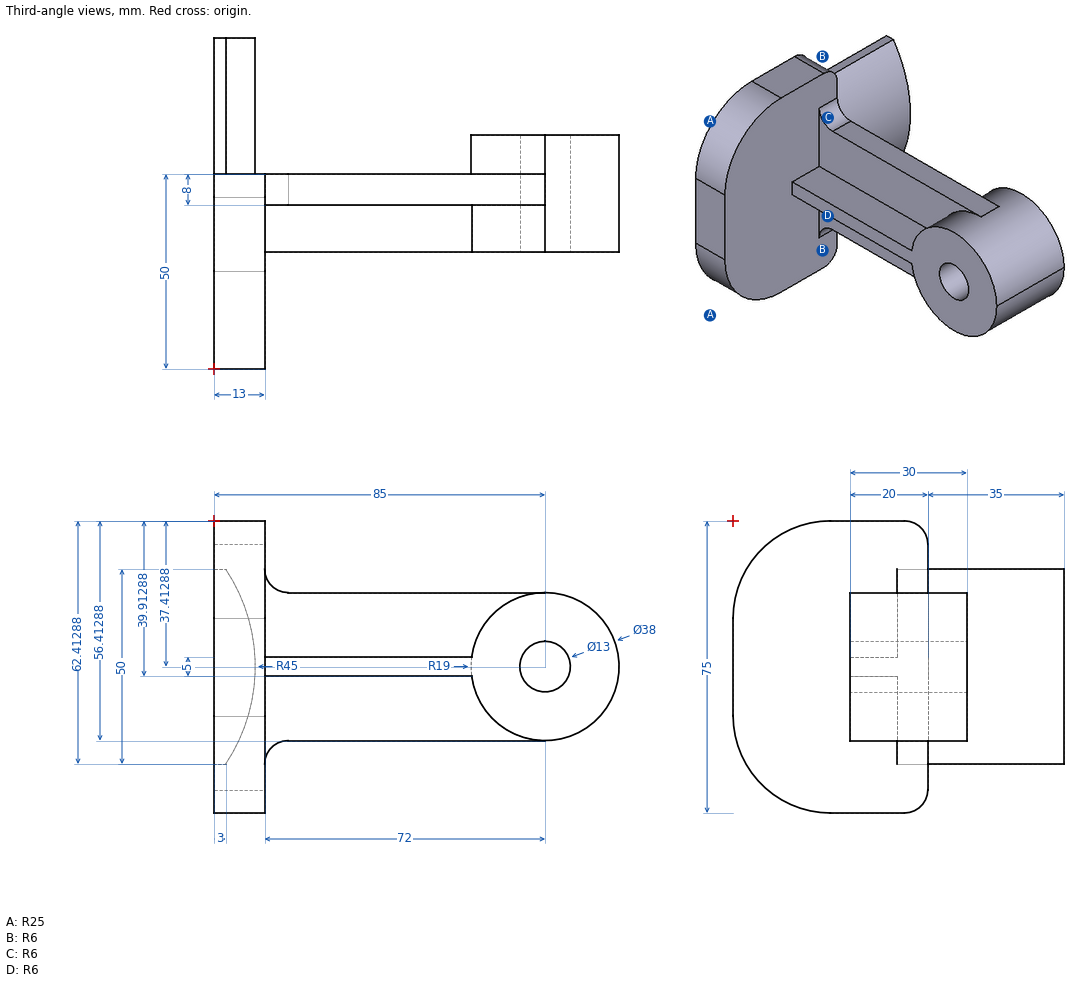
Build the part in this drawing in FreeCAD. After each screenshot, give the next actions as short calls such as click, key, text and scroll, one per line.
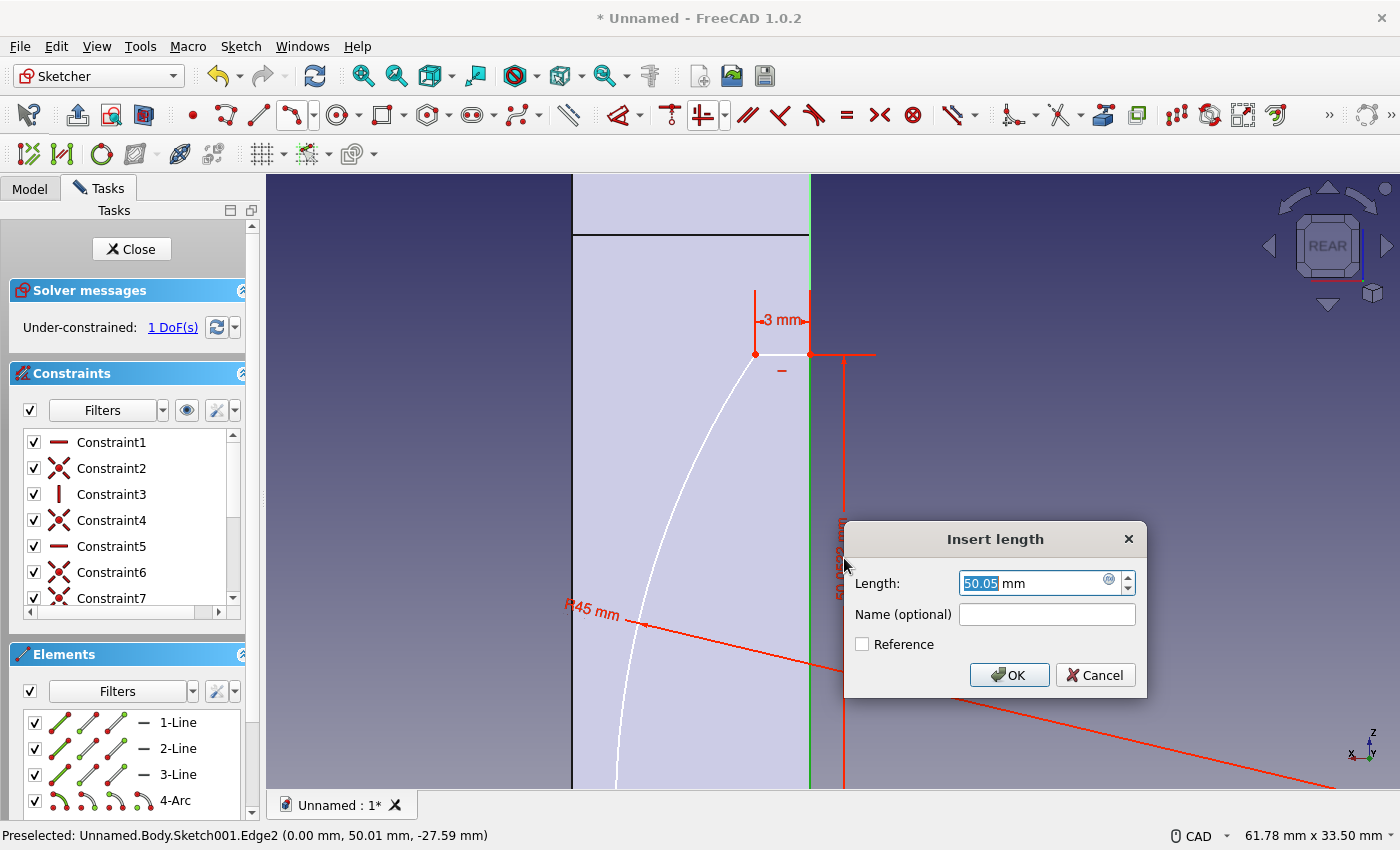
text(50)
key(Return)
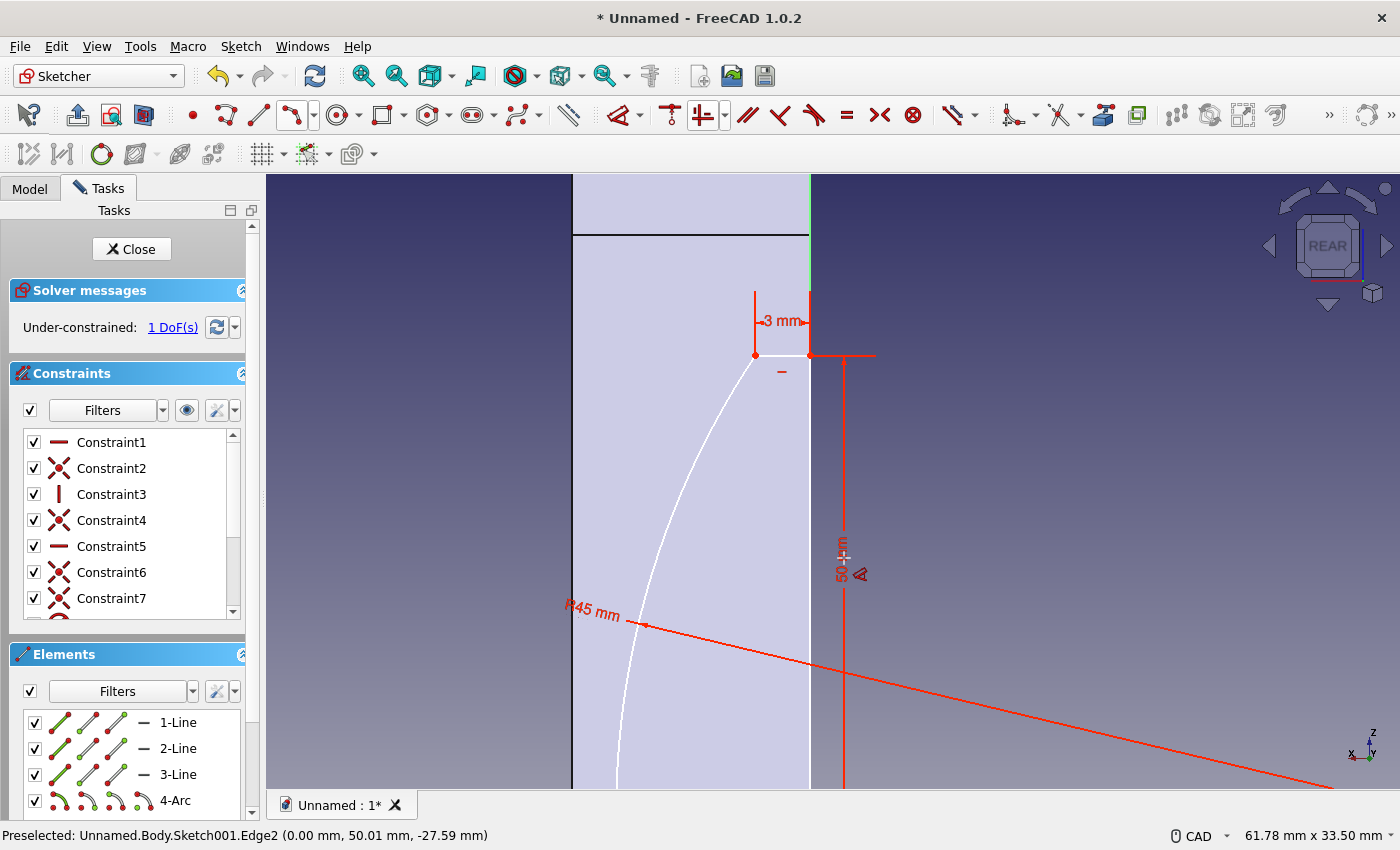
scroll(794, 356, down, 5)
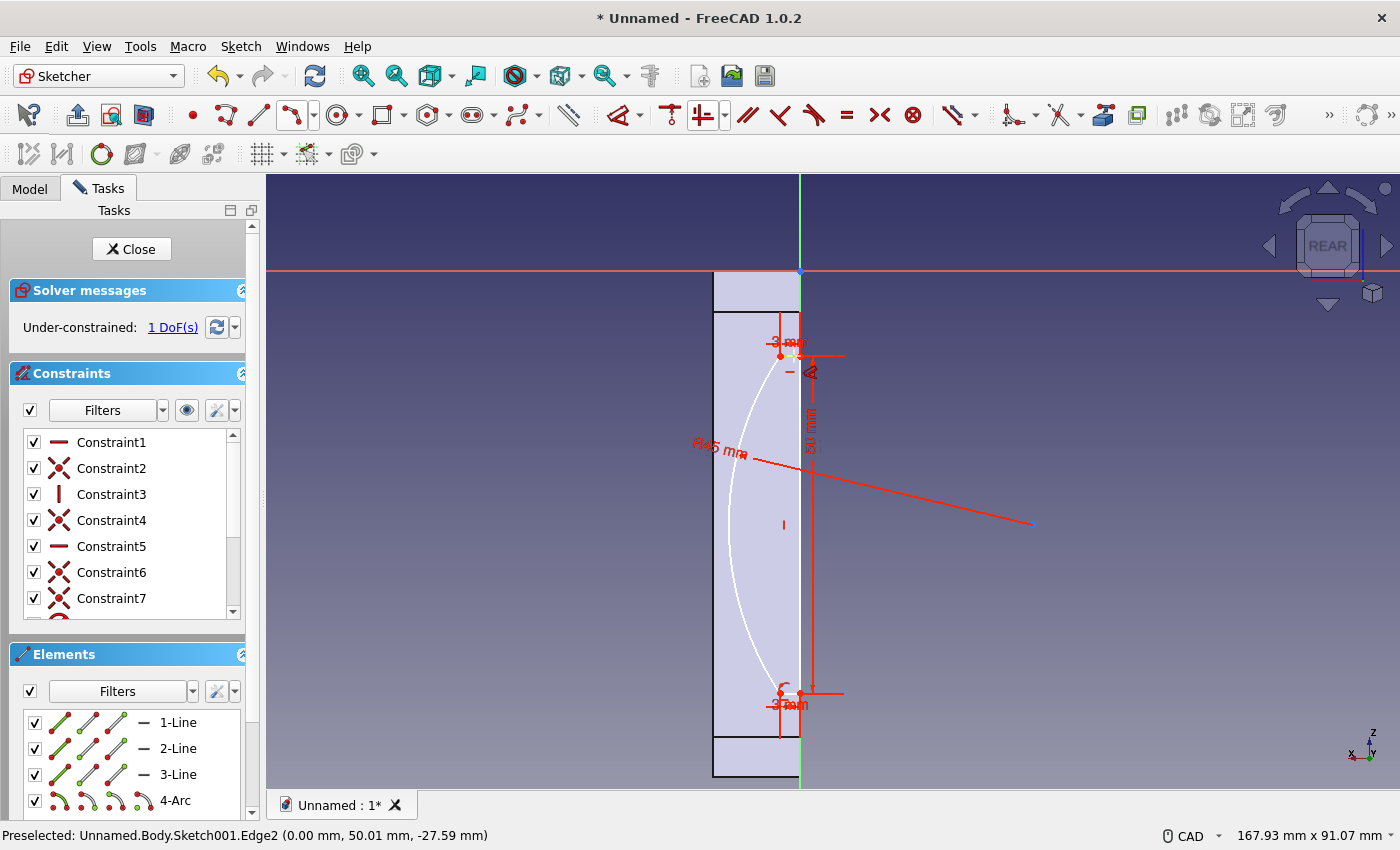
click(780, 694)
click(834, 482)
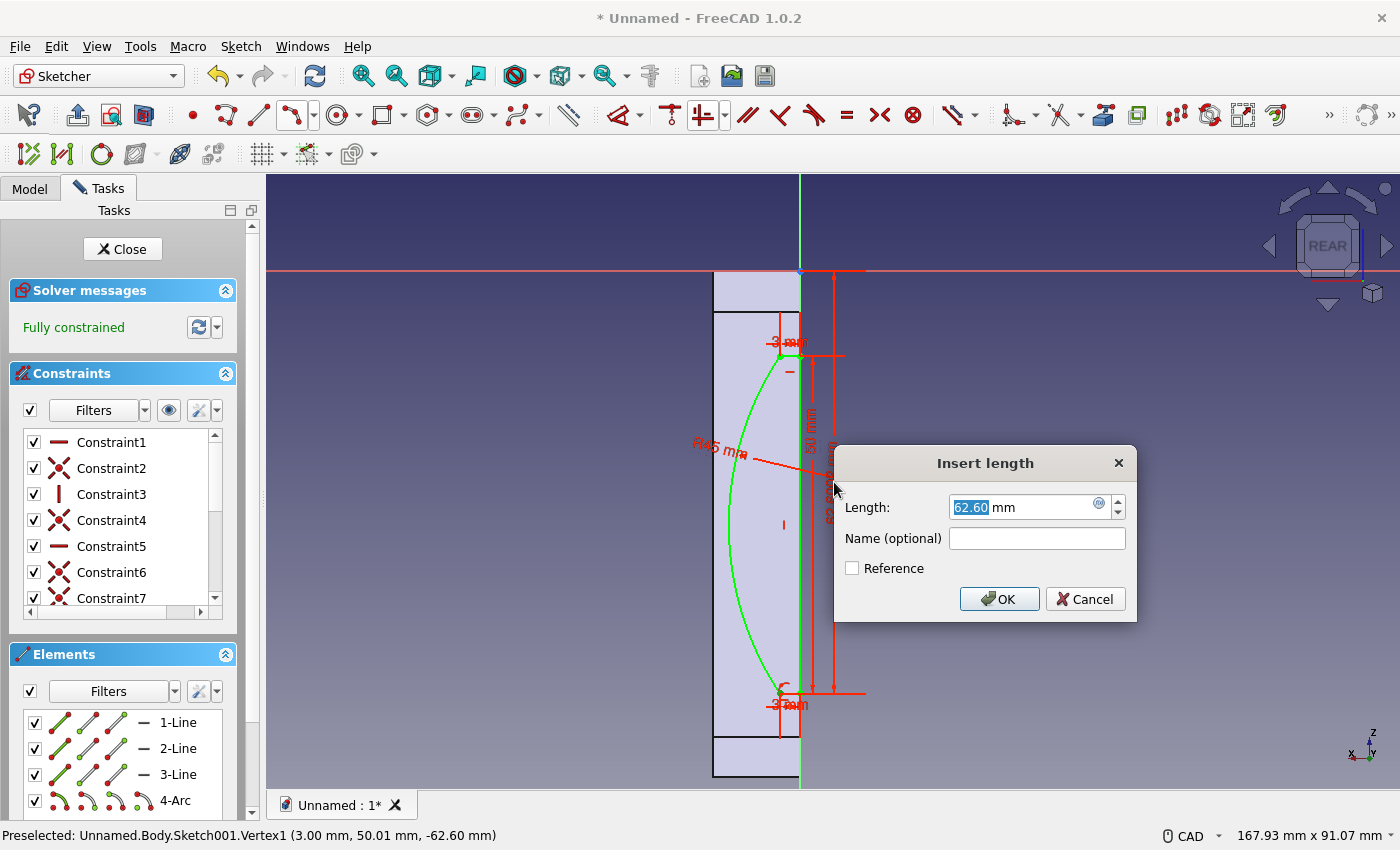
text(62.41288)
key(Return)
key(Escape)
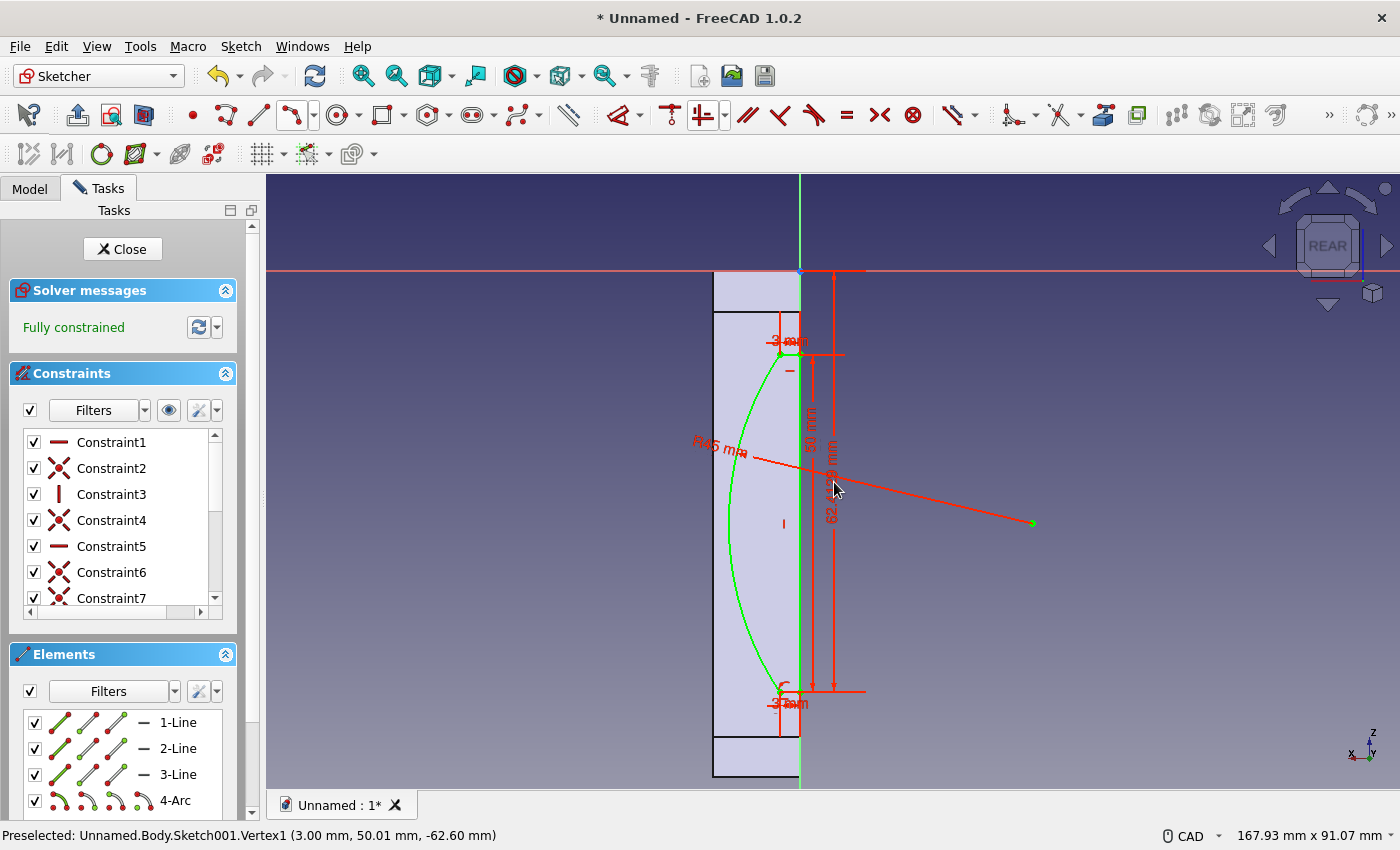
click(123, 249)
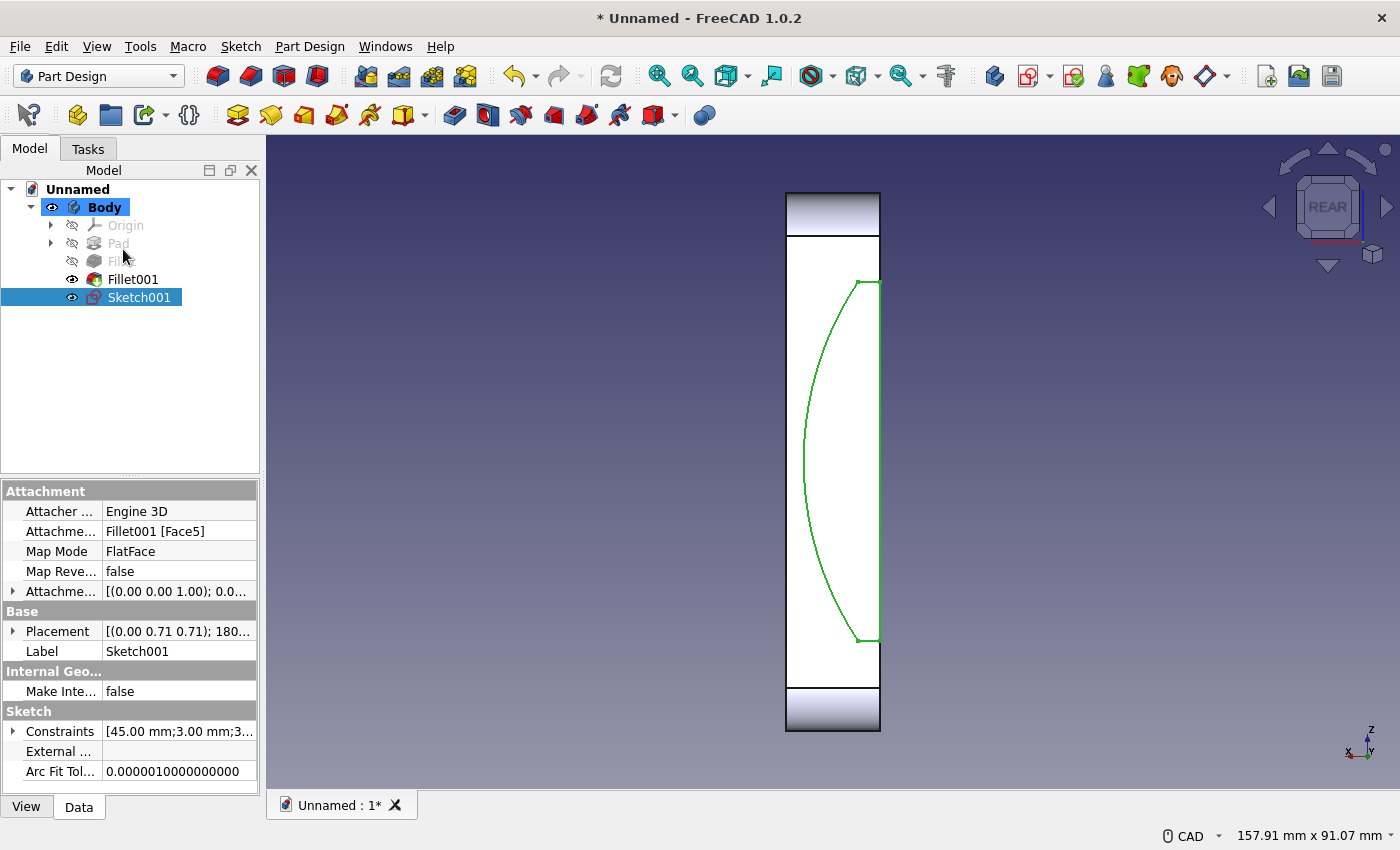
click(238, 116)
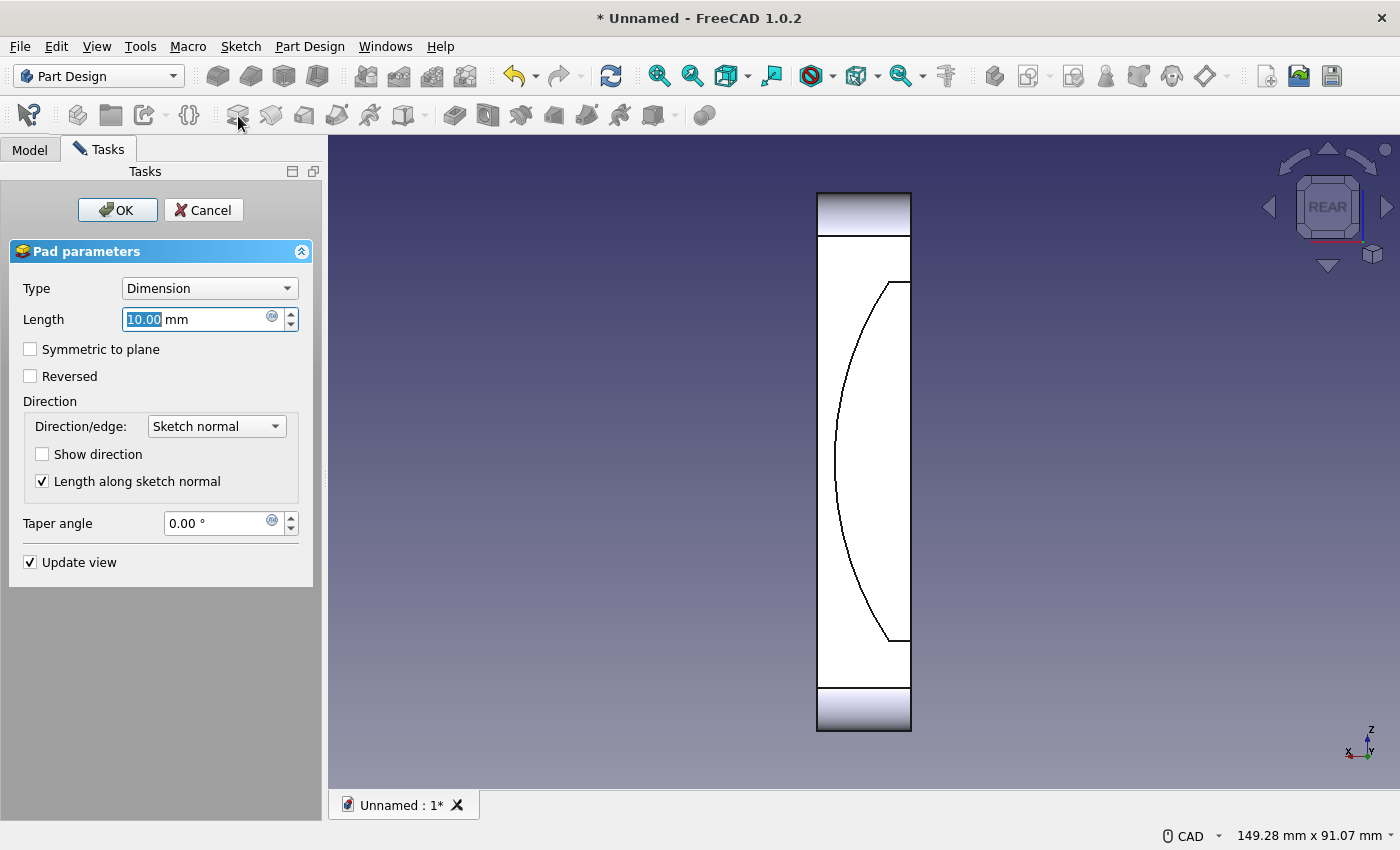
text(35)
key(Tab)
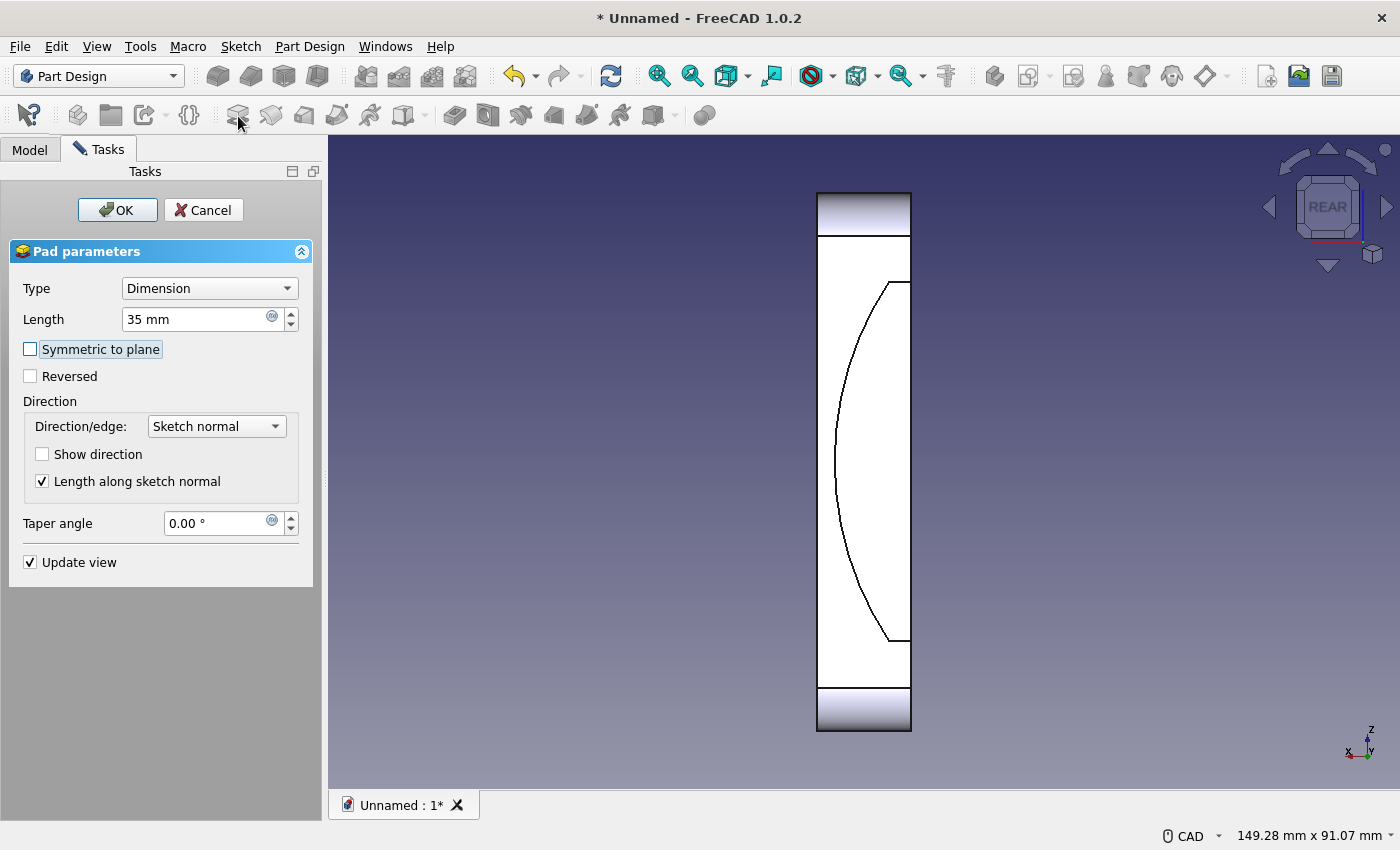
click(118, 210)